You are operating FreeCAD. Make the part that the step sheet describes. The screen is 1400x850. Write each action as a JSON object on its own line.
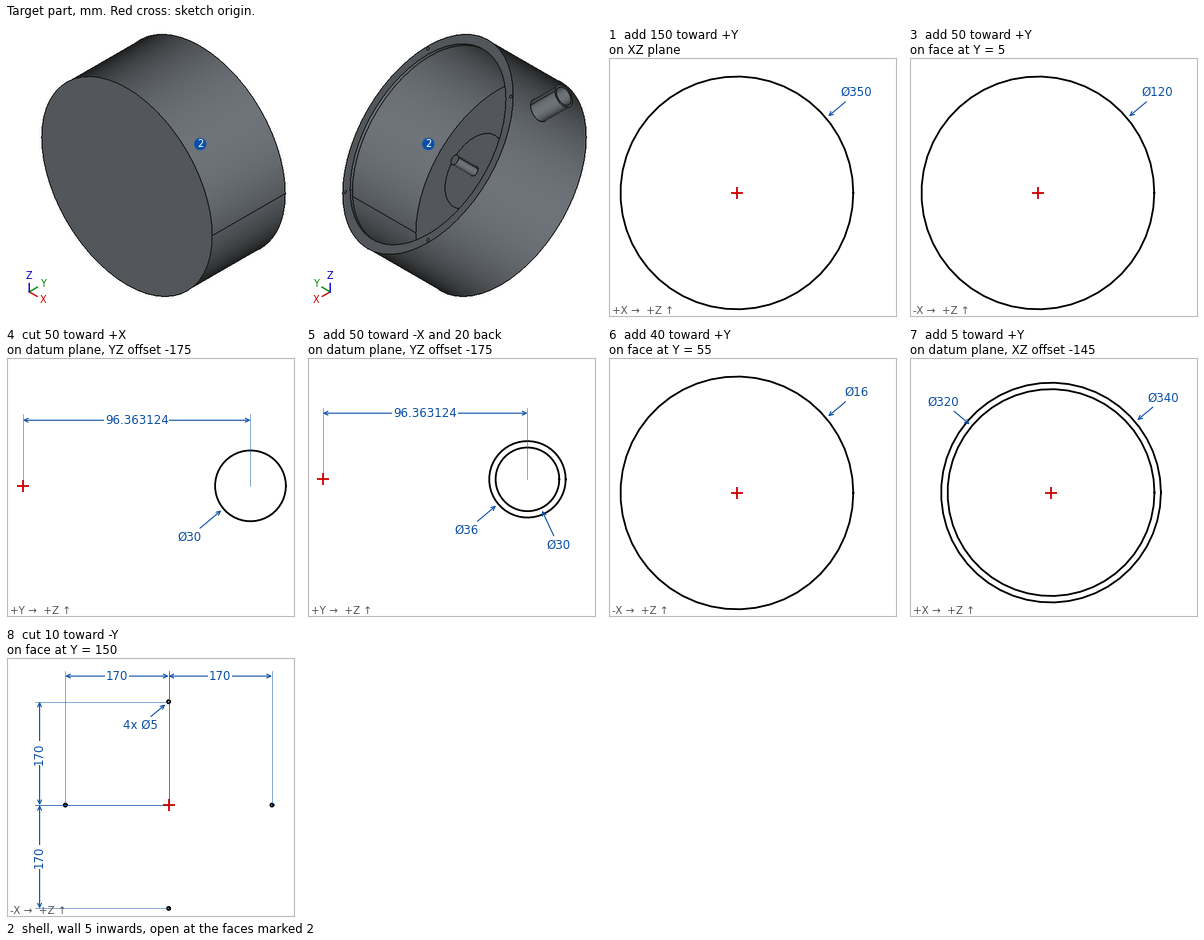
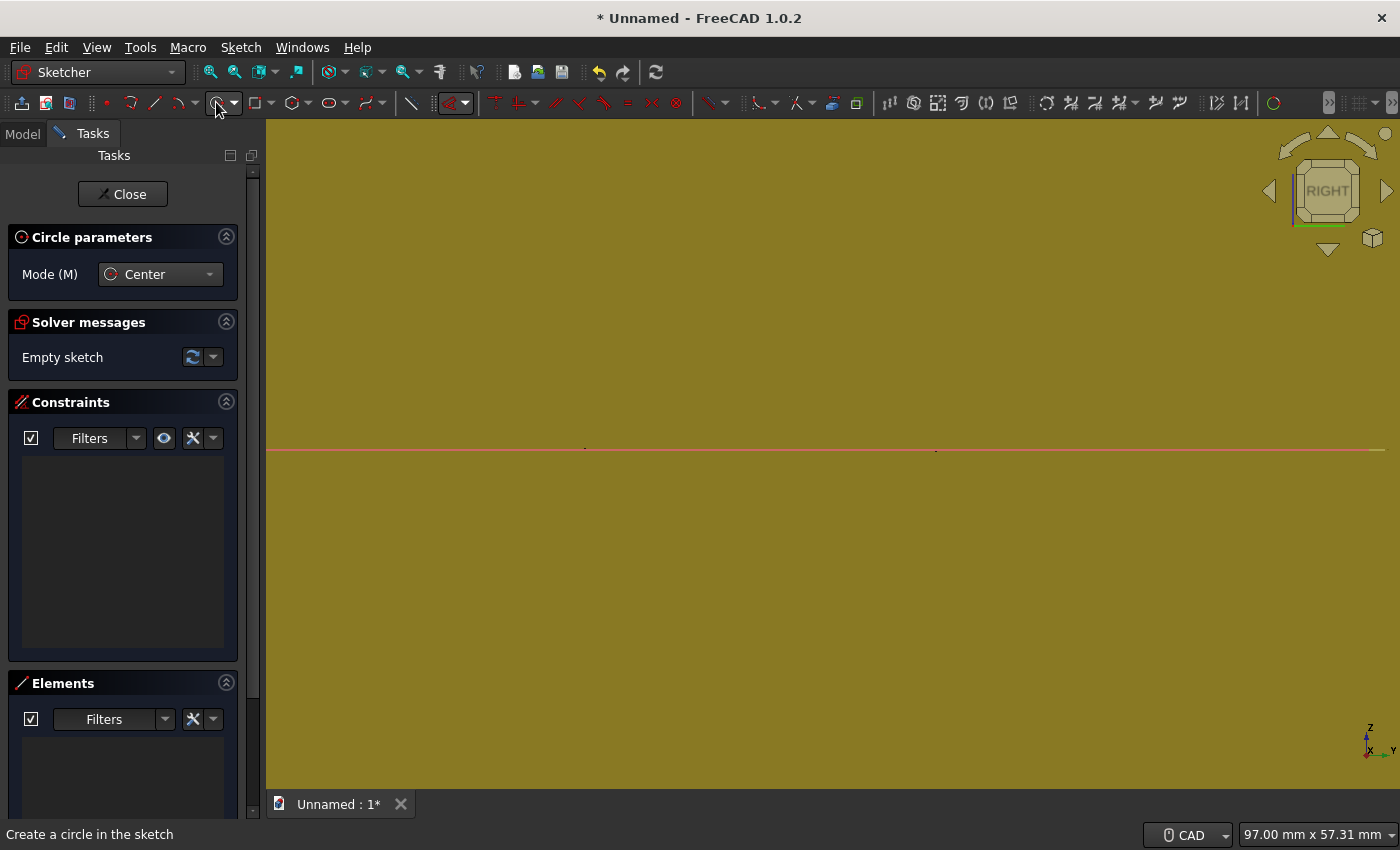
{"action": "left_click", "coordinate": [760, 450]}
{"action": "mouse_move", "coordinate": [909, 301]}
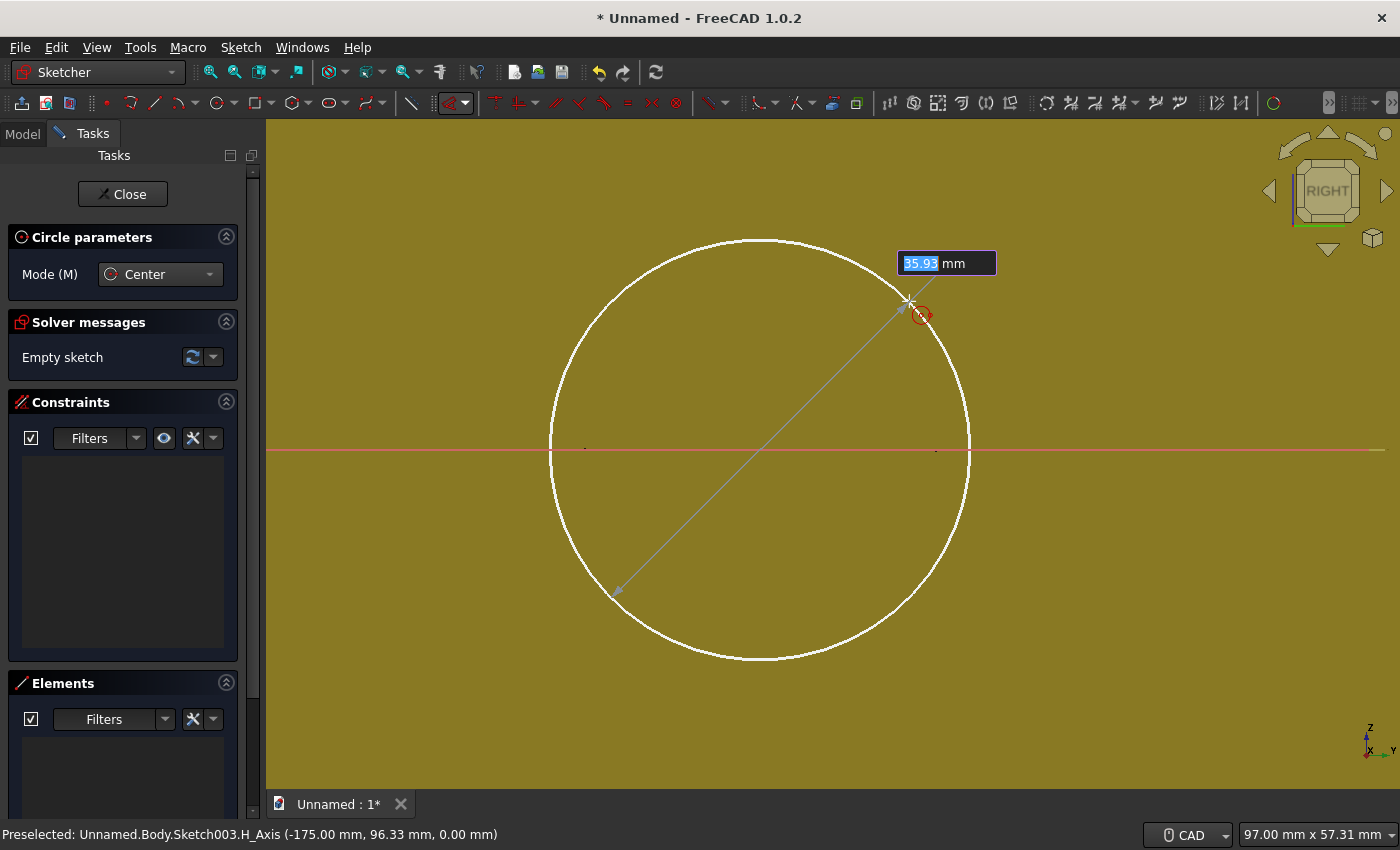
{"action": "type", "text": "36"}
{"action": "key", "text": "Return"}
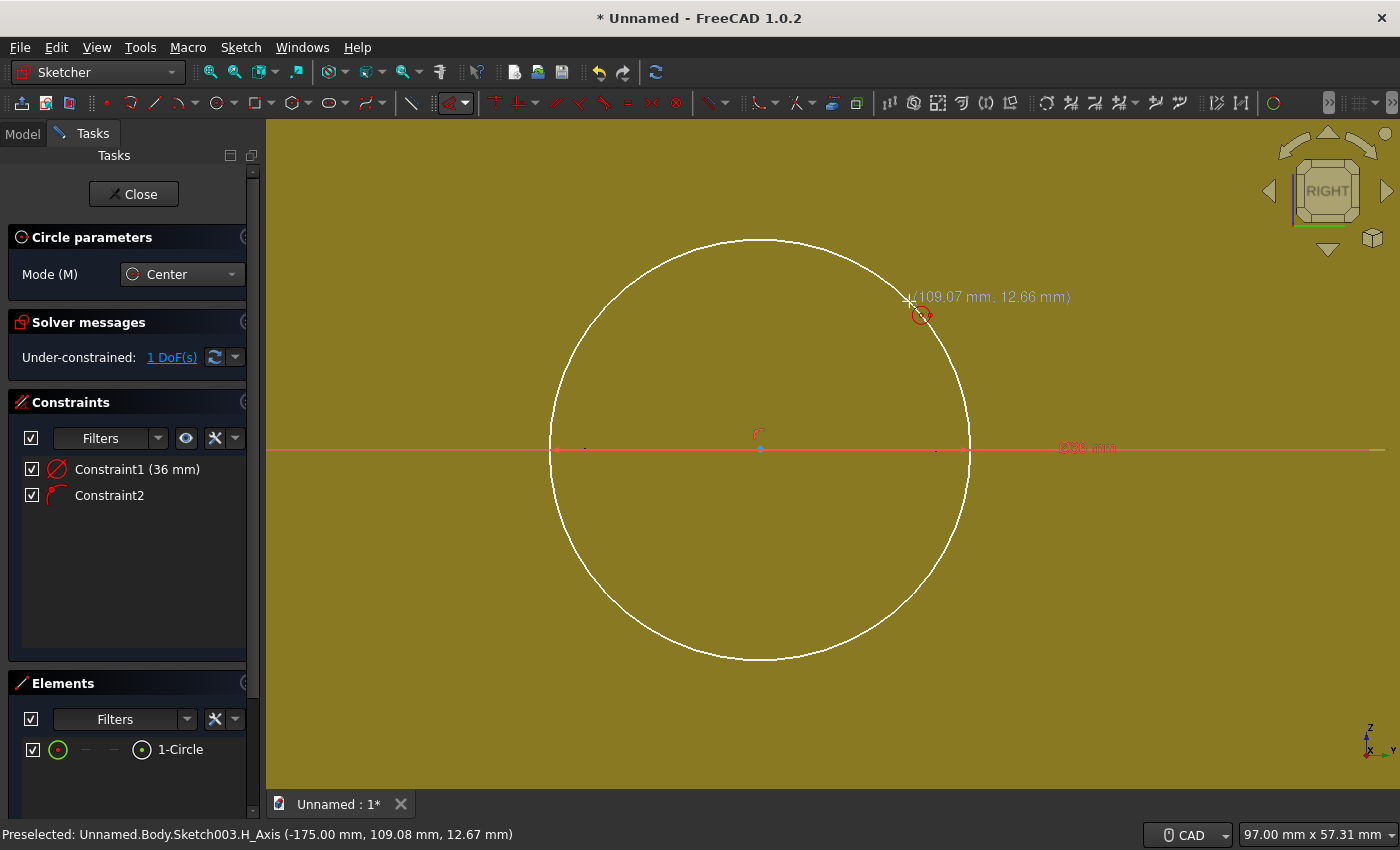
{"action": "left_click", "coordinate": [760, 450]}
{"action": "mouse_move", "coordinate": [884, 326]}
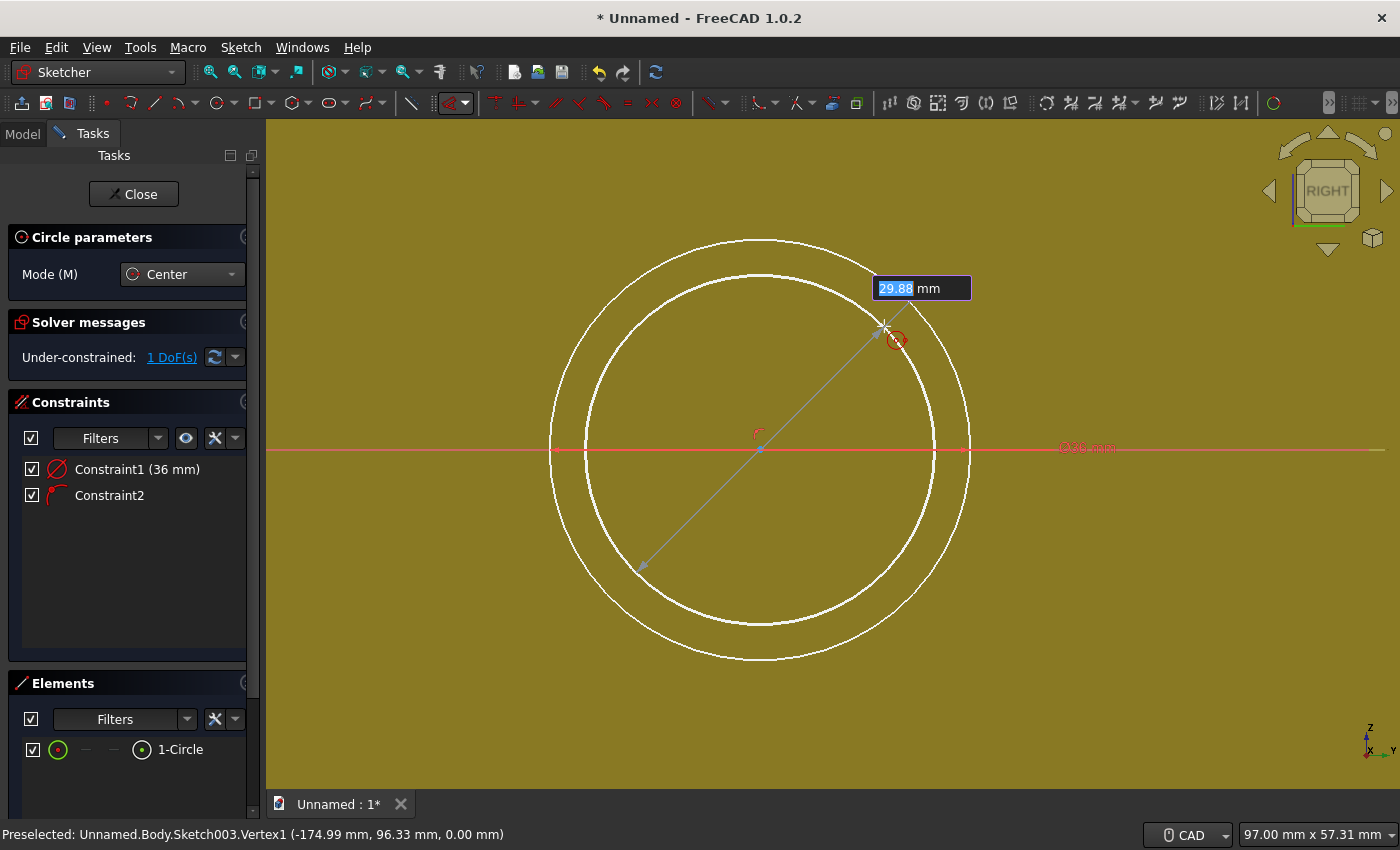
{"action": "type", "text": "30"}
{"action": "key", "text": "Return"}
{"action": "key", "text": "Escape"}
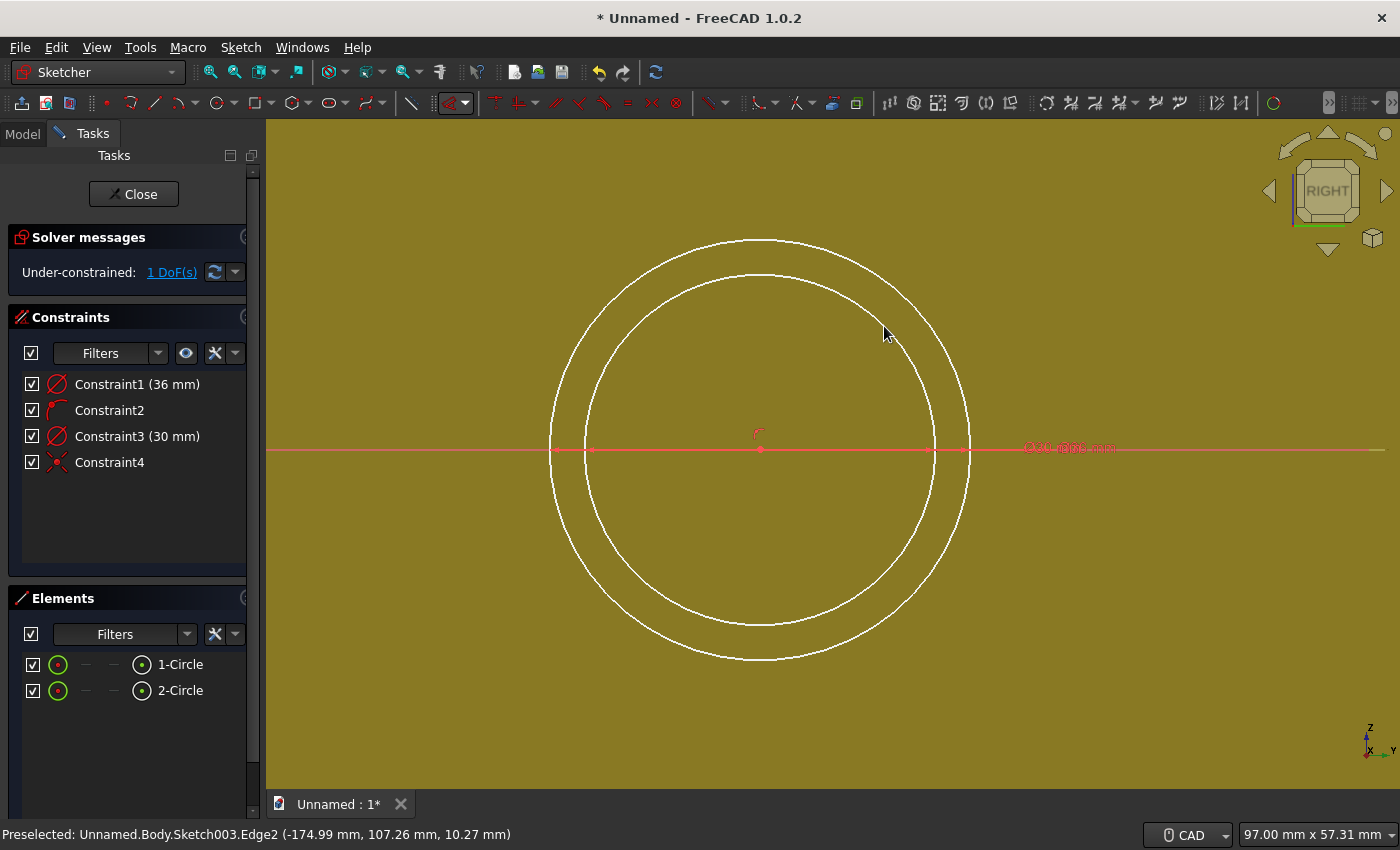
{"action": "left_click", "coordinate": [760, 450]}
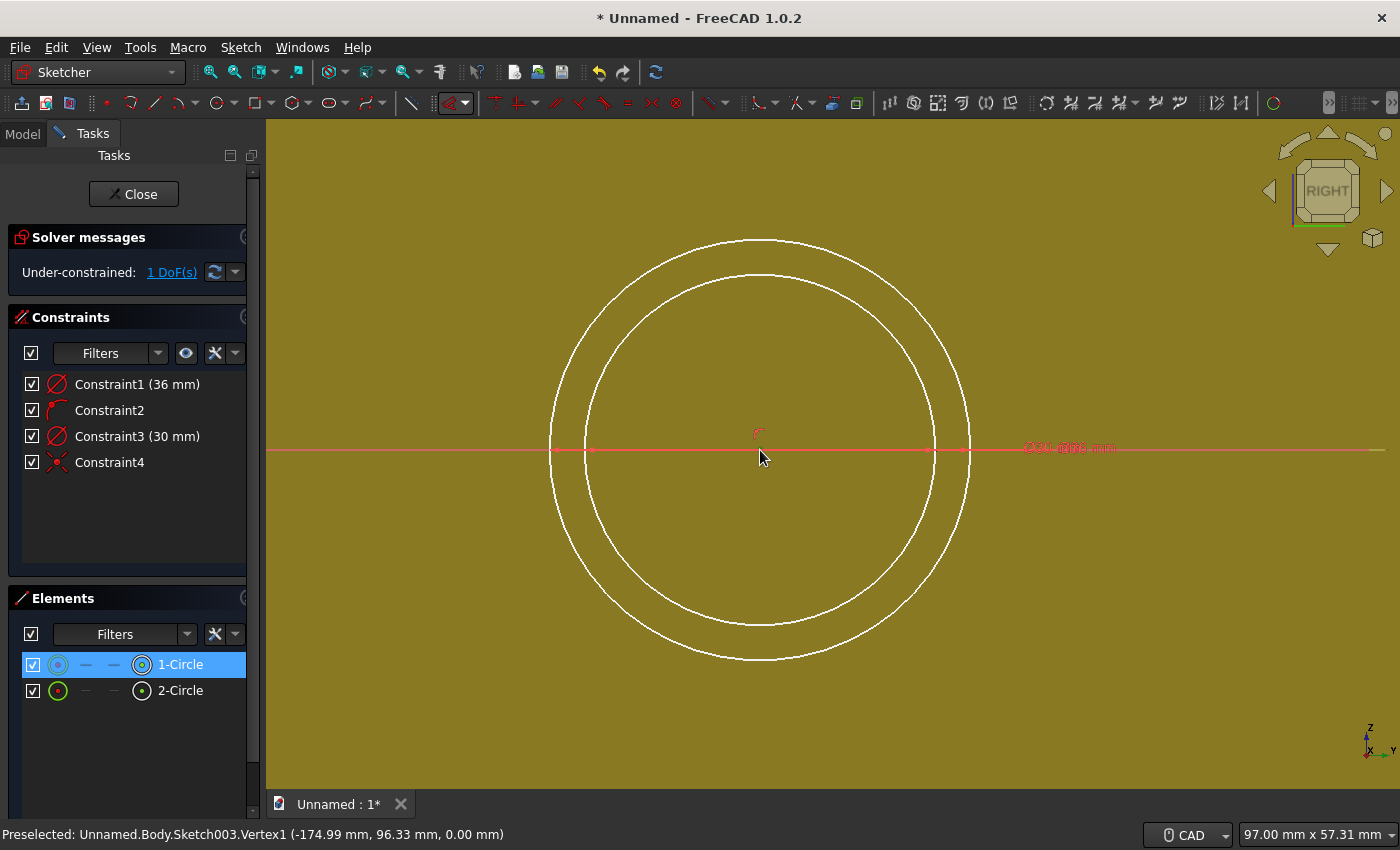
{"action": "left_click", "coordinate": [468, 104]}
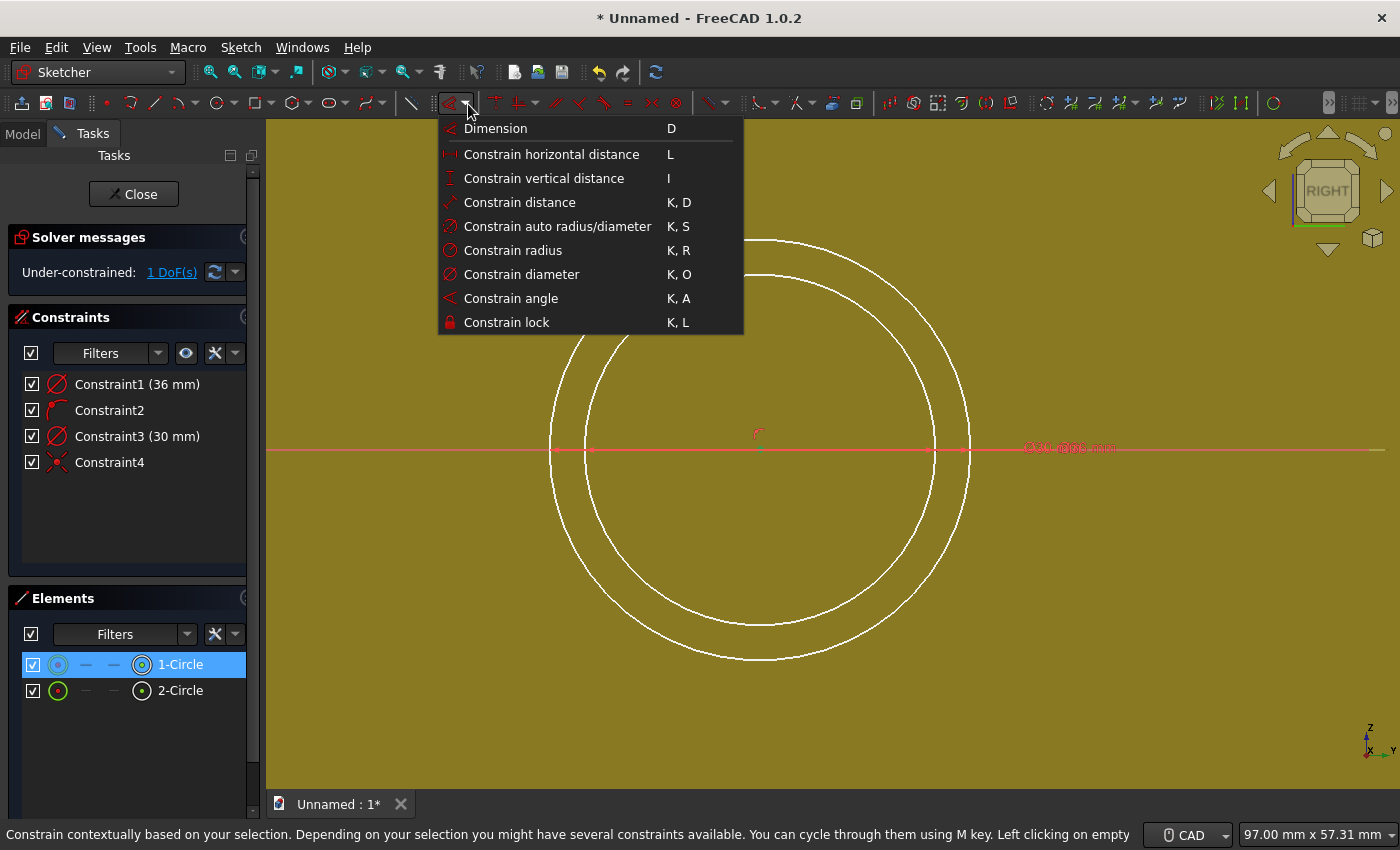
{"action": "left_click", "coordinate": [591, 154]}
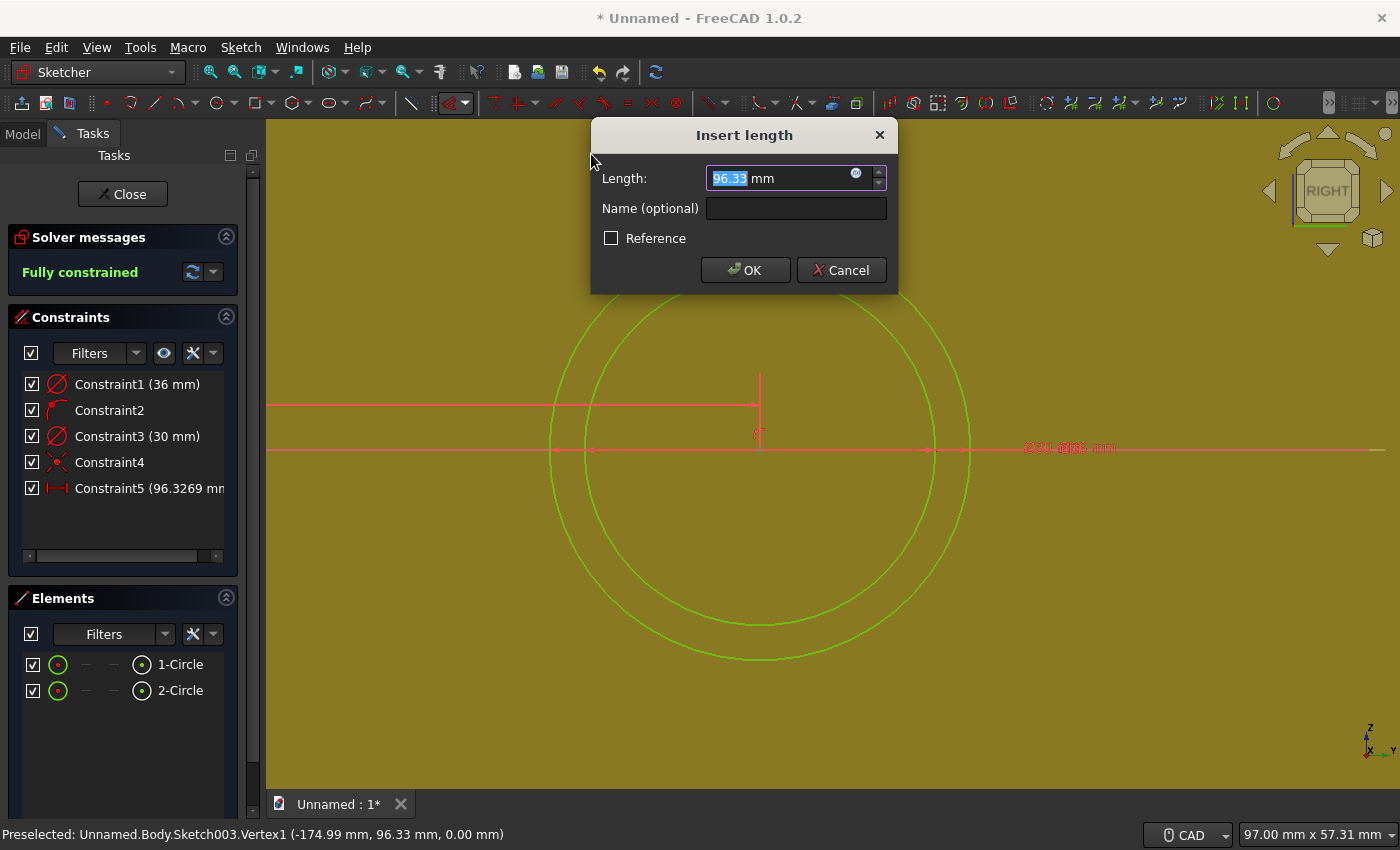
{"action": "type", "text": "96.363124"}
{"action": "key", "text": "Return"}